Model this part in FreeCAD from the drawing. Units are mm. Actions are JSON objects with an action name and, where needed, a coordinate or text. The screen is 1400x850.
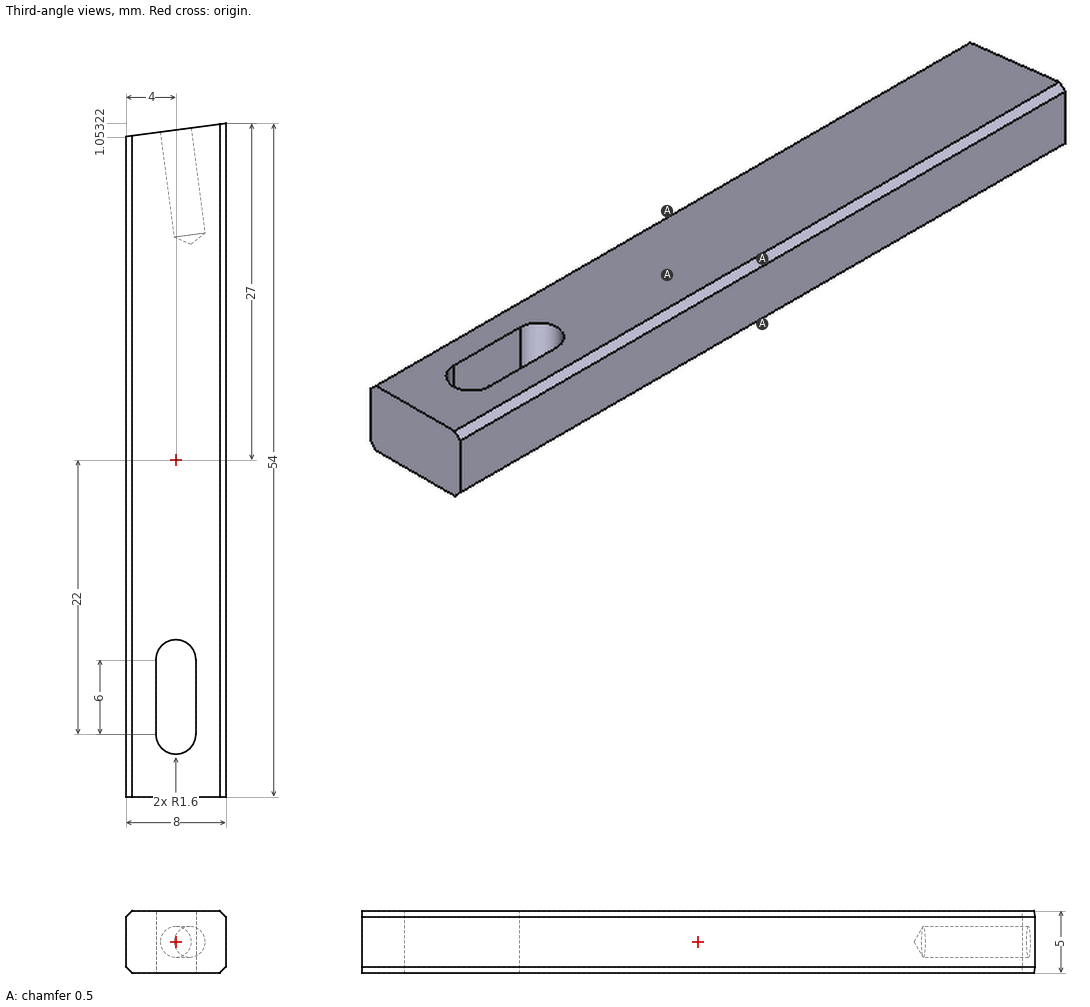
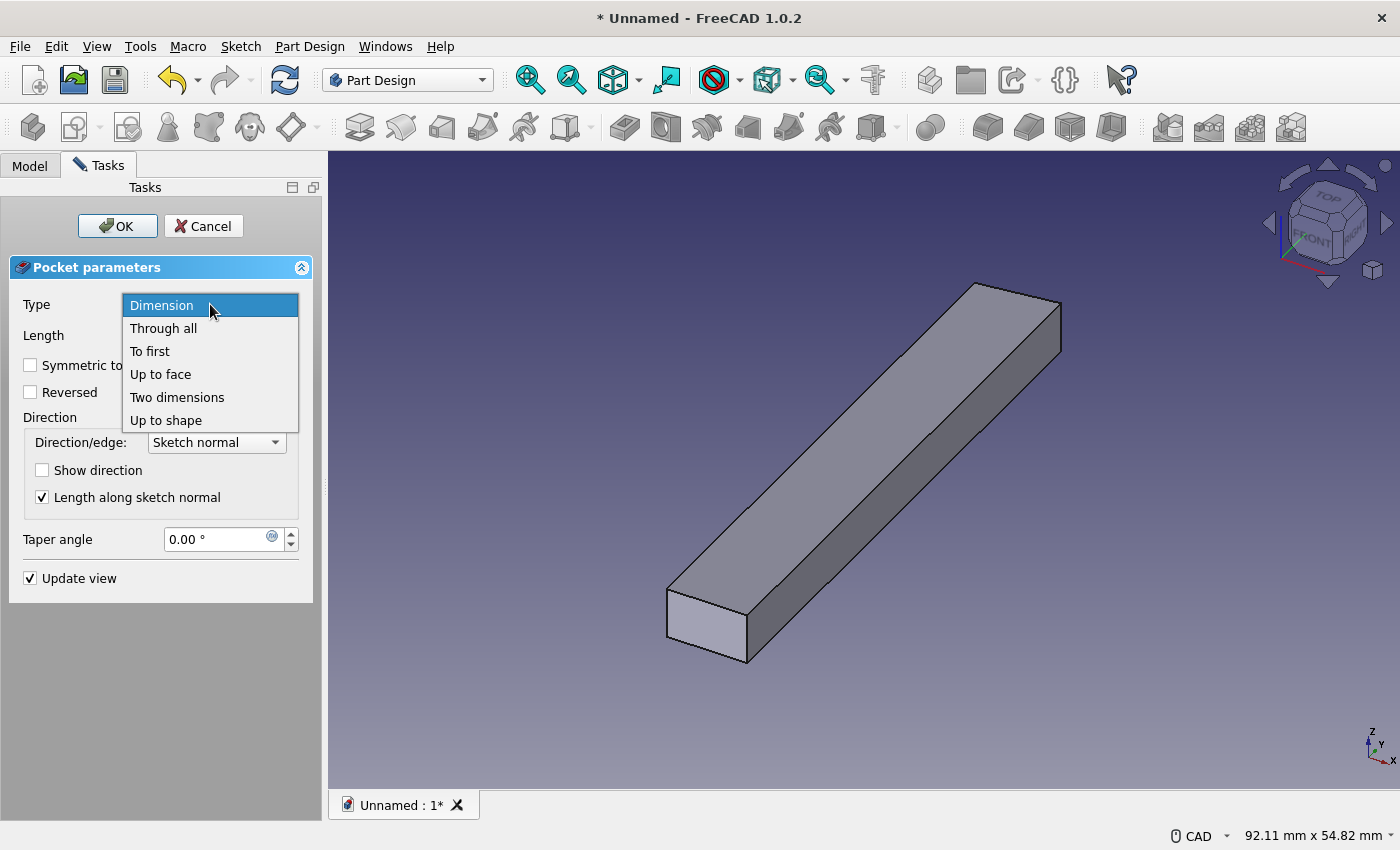
{"action": "left_click", "coordinate": [208, 328]}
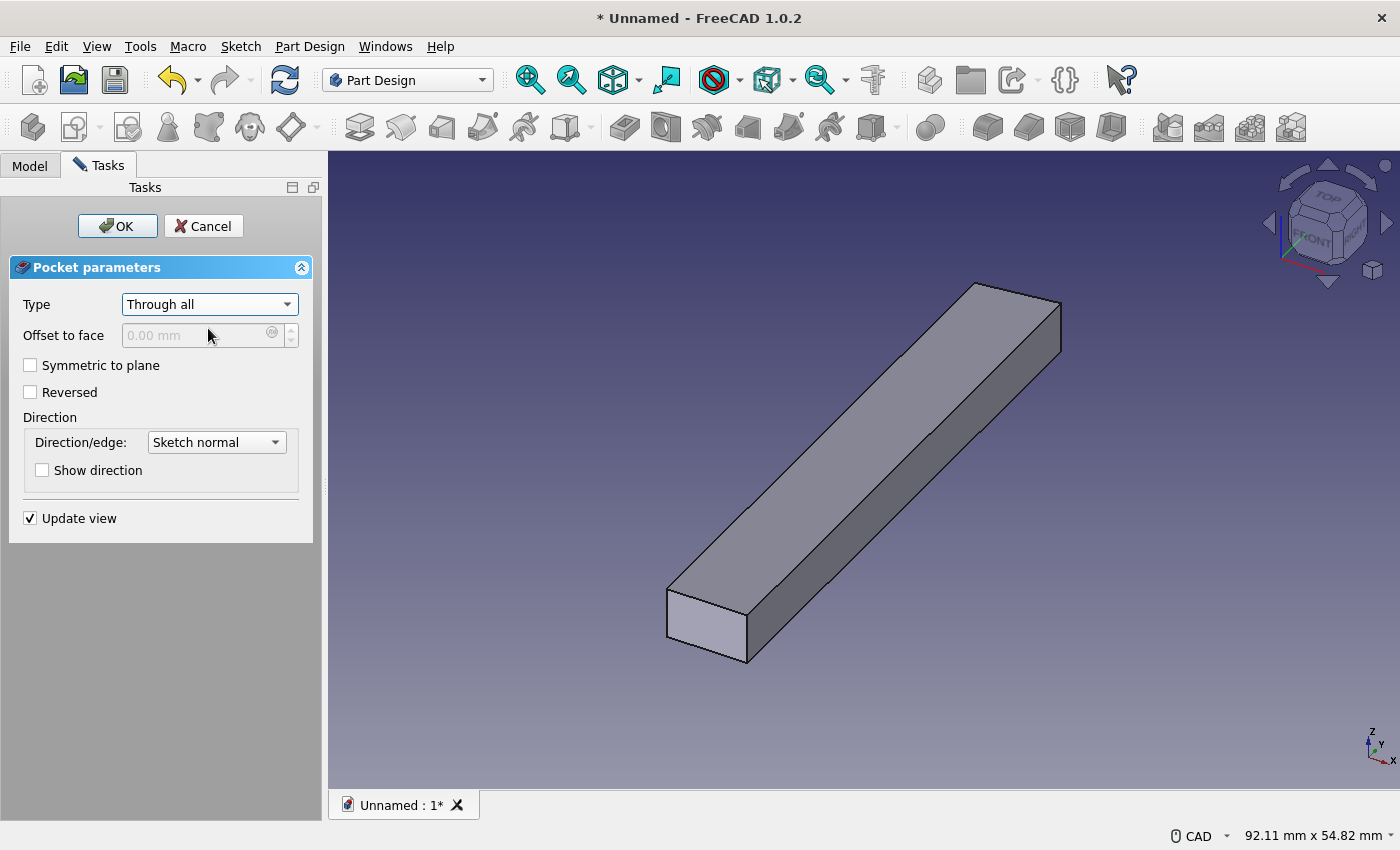
{"action": "left_click", "coordinate": [118, 226]}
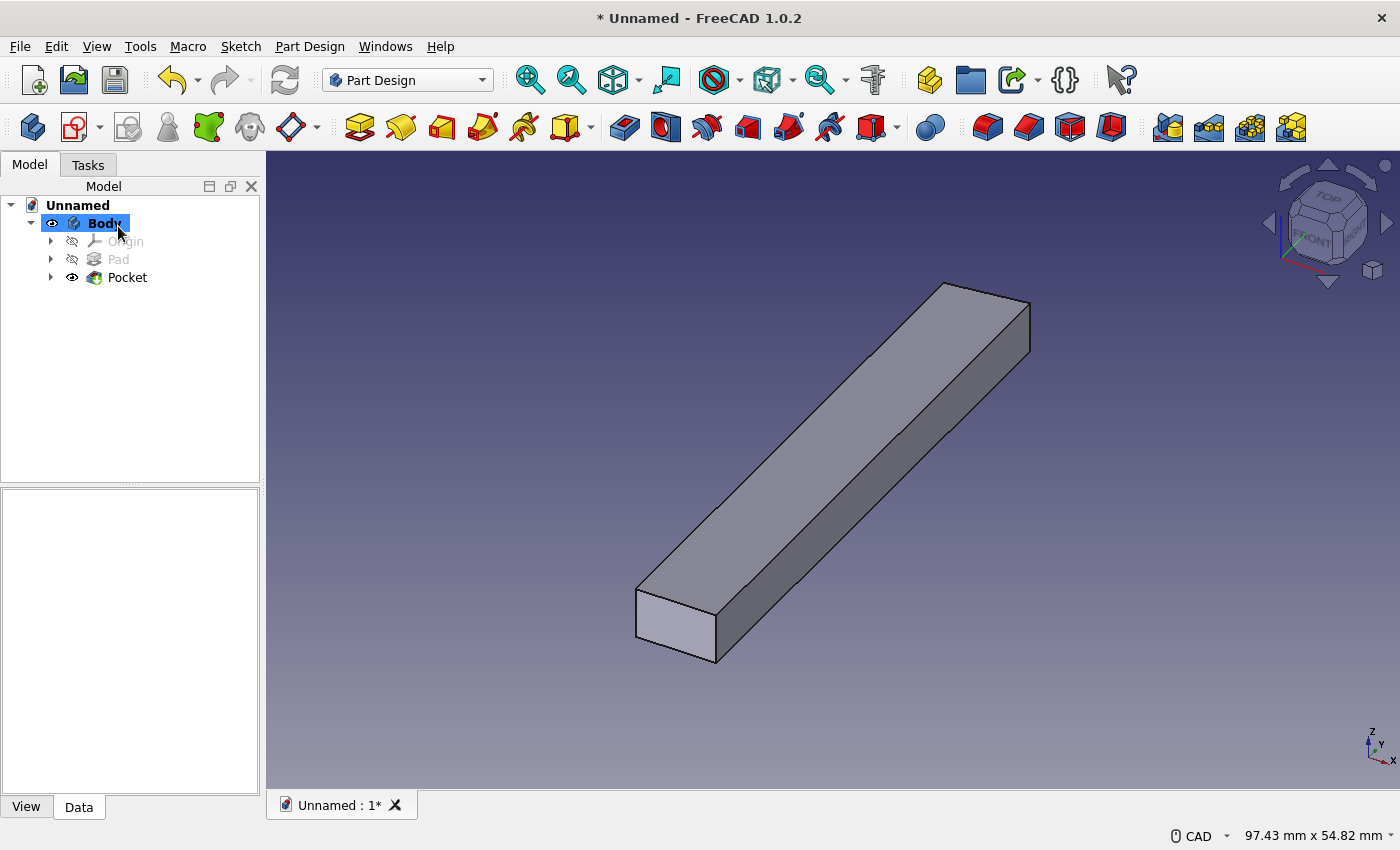
{"action": "key", "text": "4"}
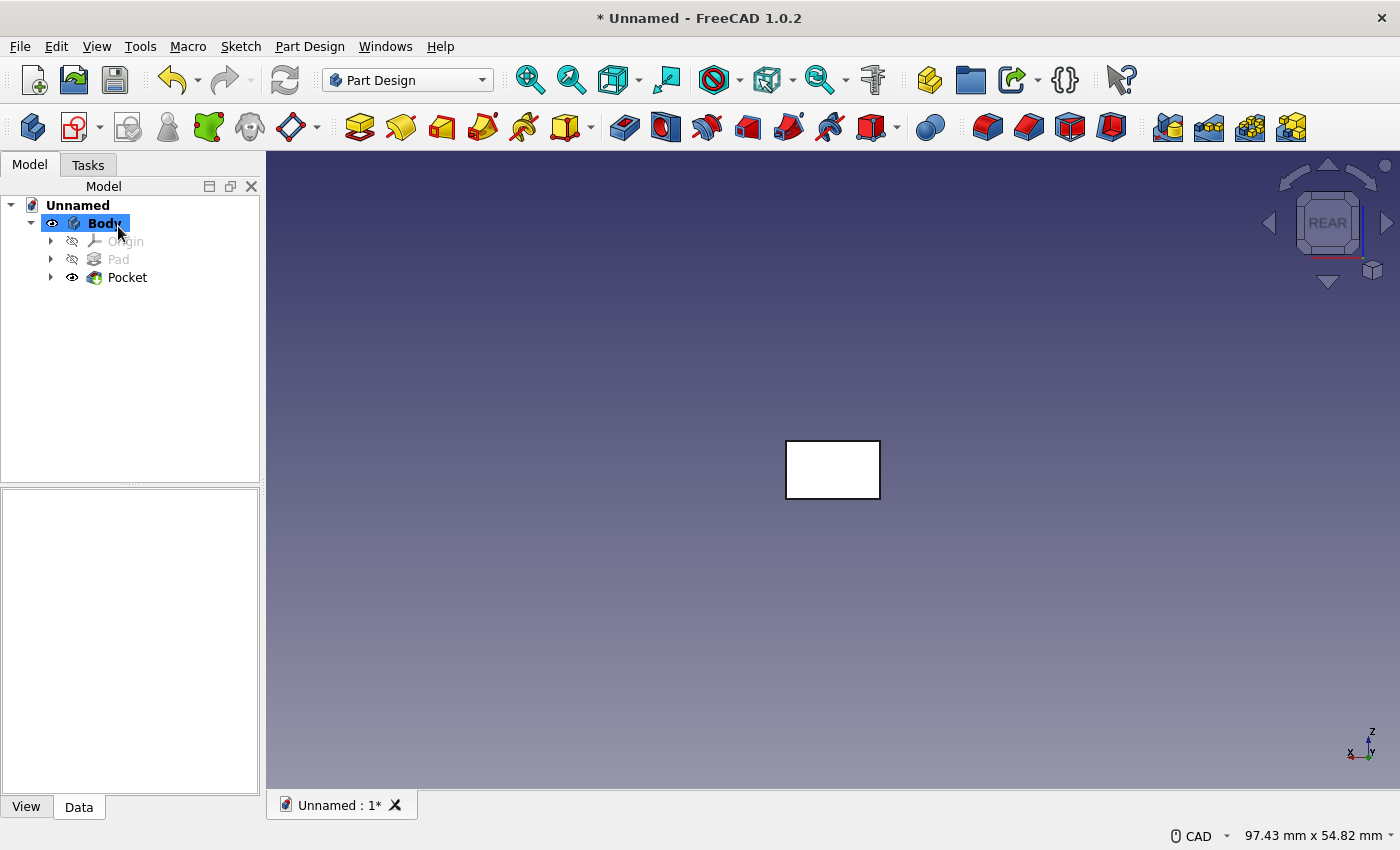
{"action": "key", "text": "v f"}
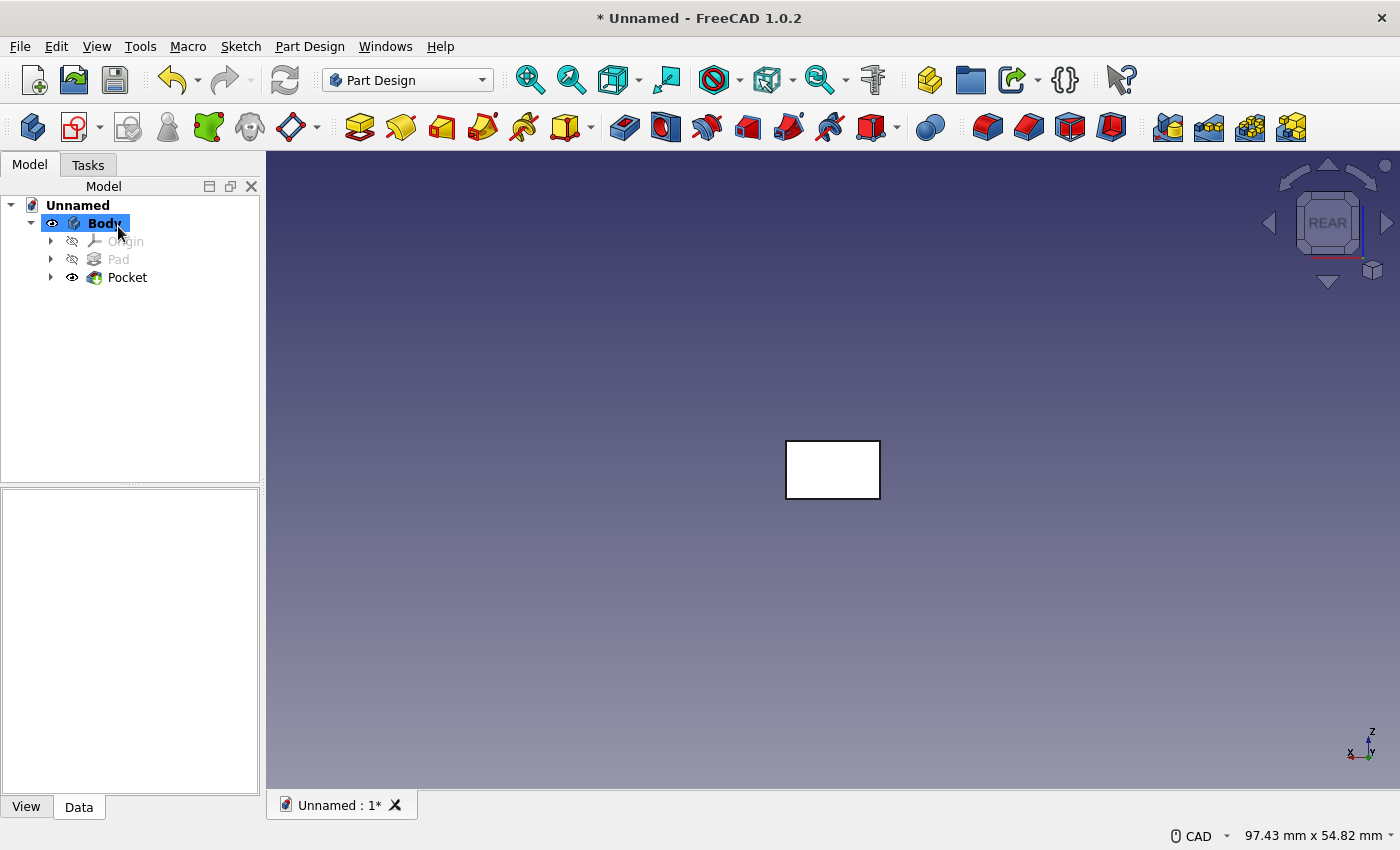
{"action": "left_click", "coordinate": [820, 469]}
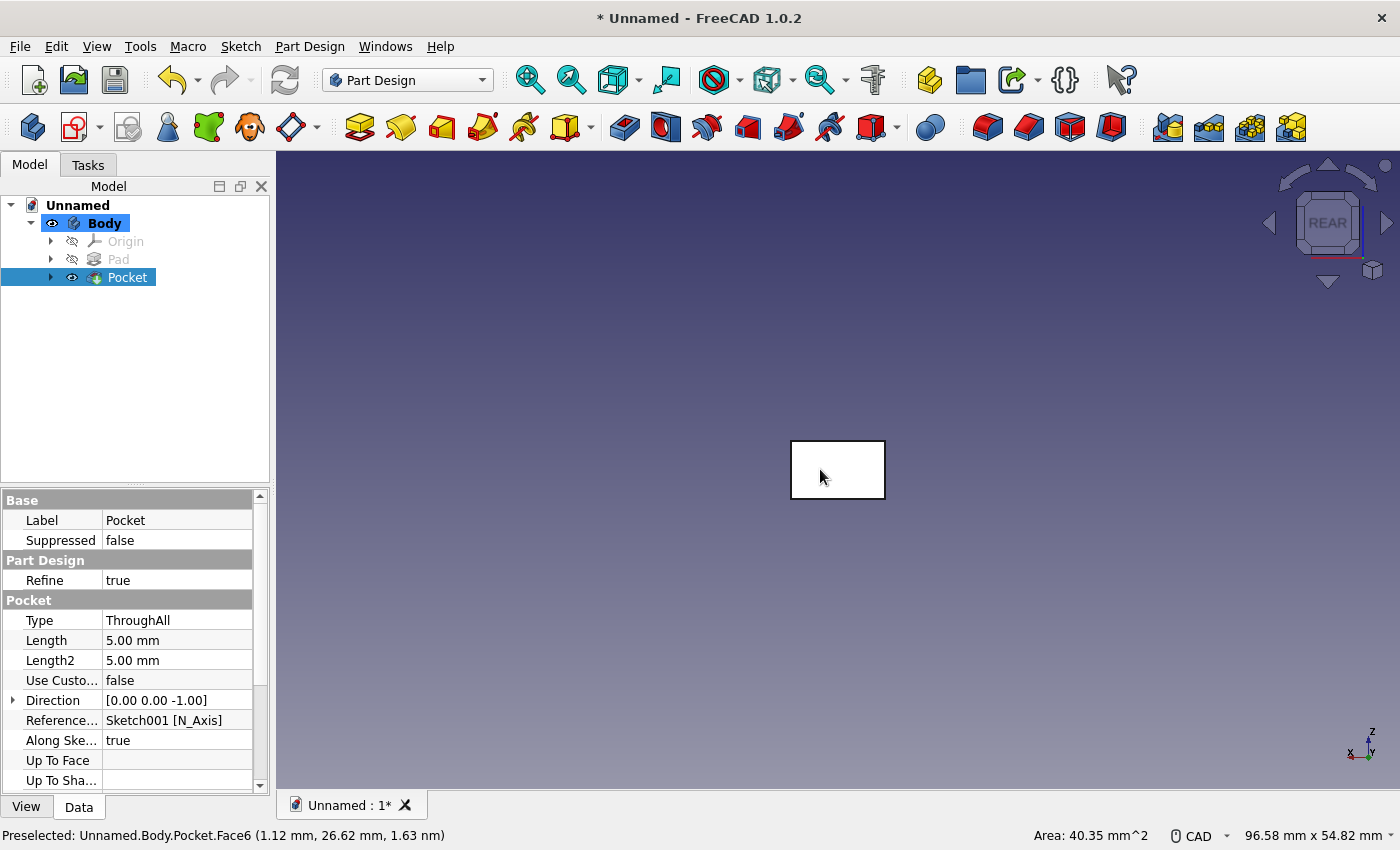
{"action": "left_click", "coordinate": [74, 128]}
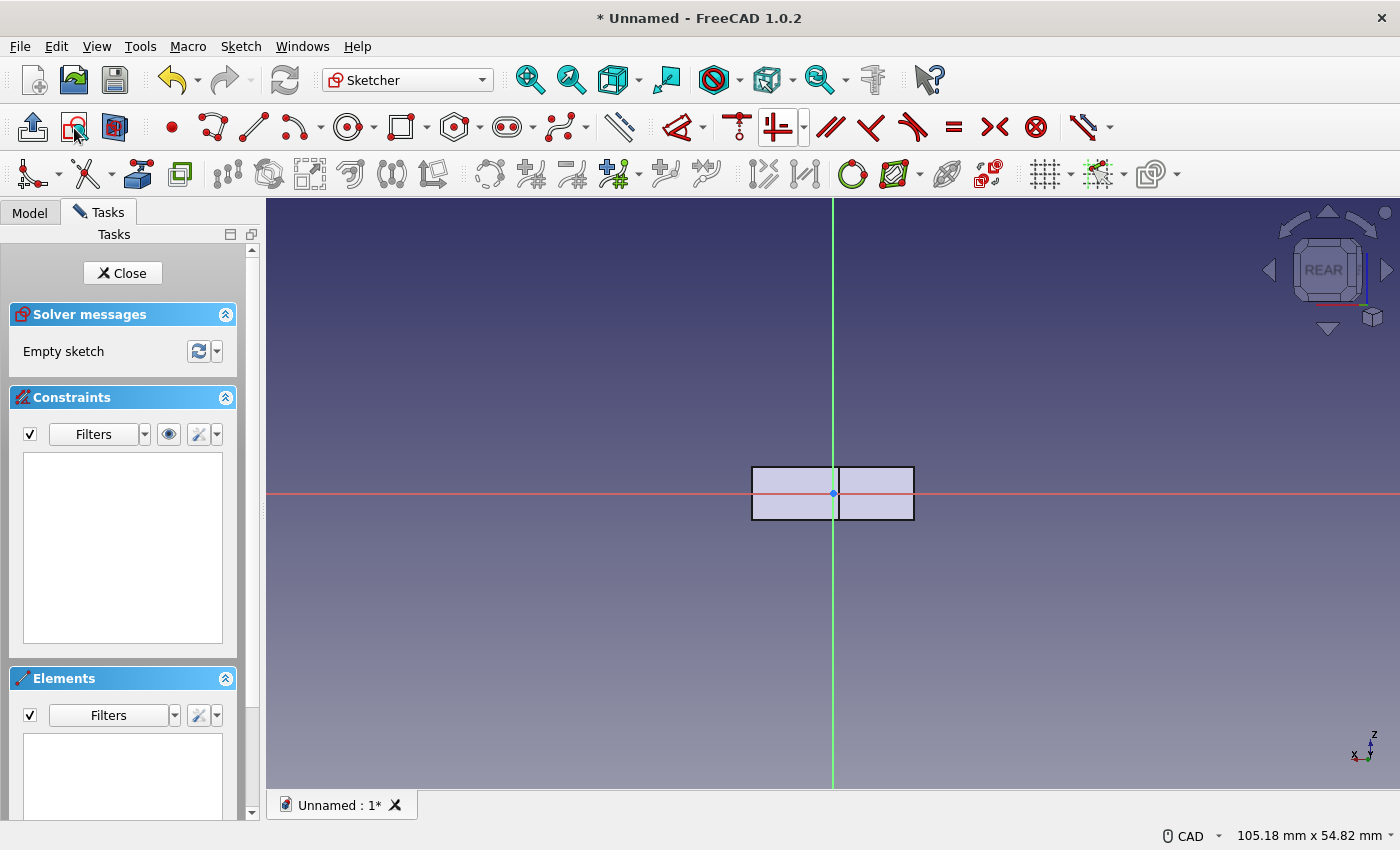
{"action": "scroll", "coordinate": [811, 494], "scroll_direction": "up", "scroll_amount": 13}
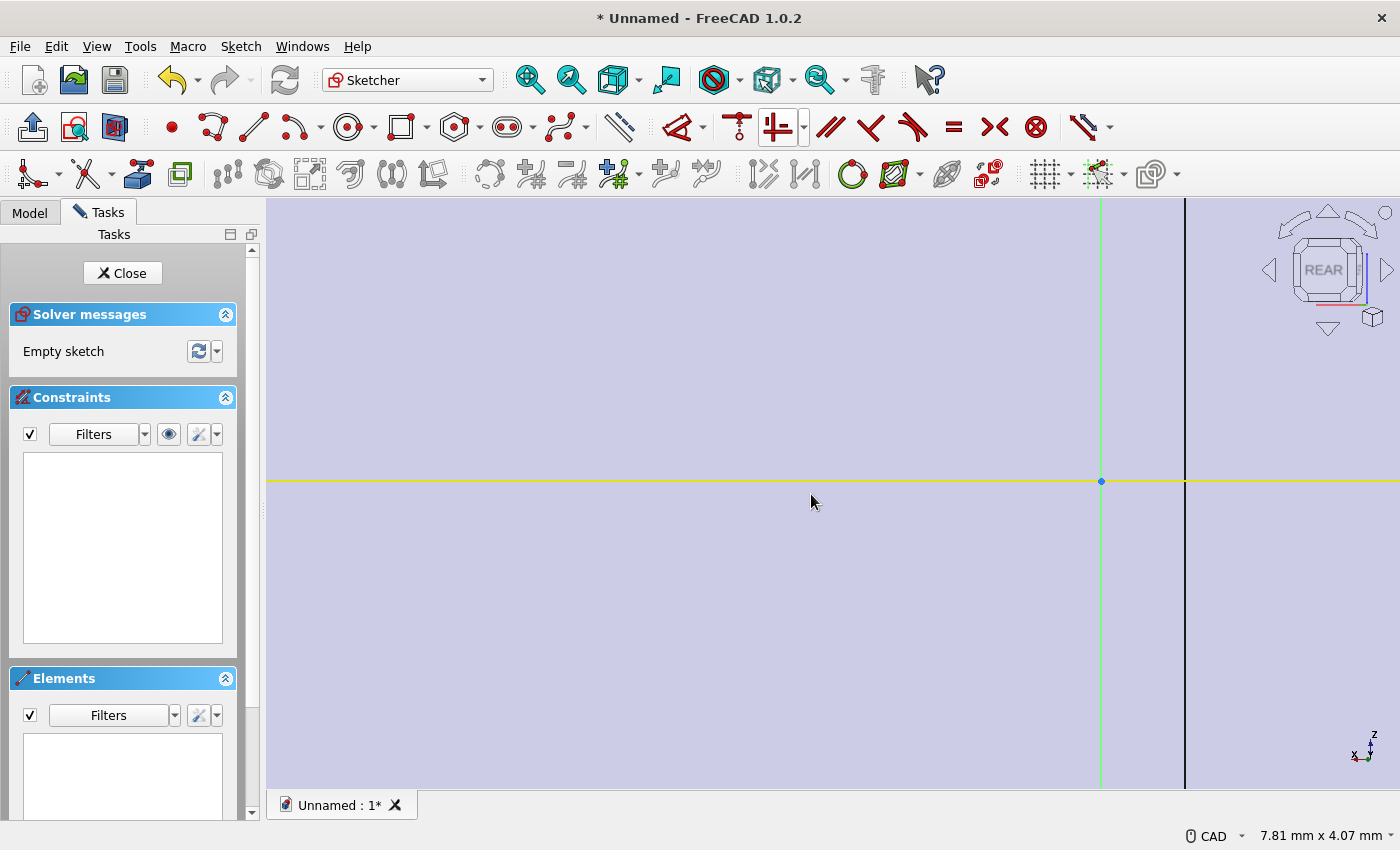
{"action": "left_click", "coordinate": [348, 128]}